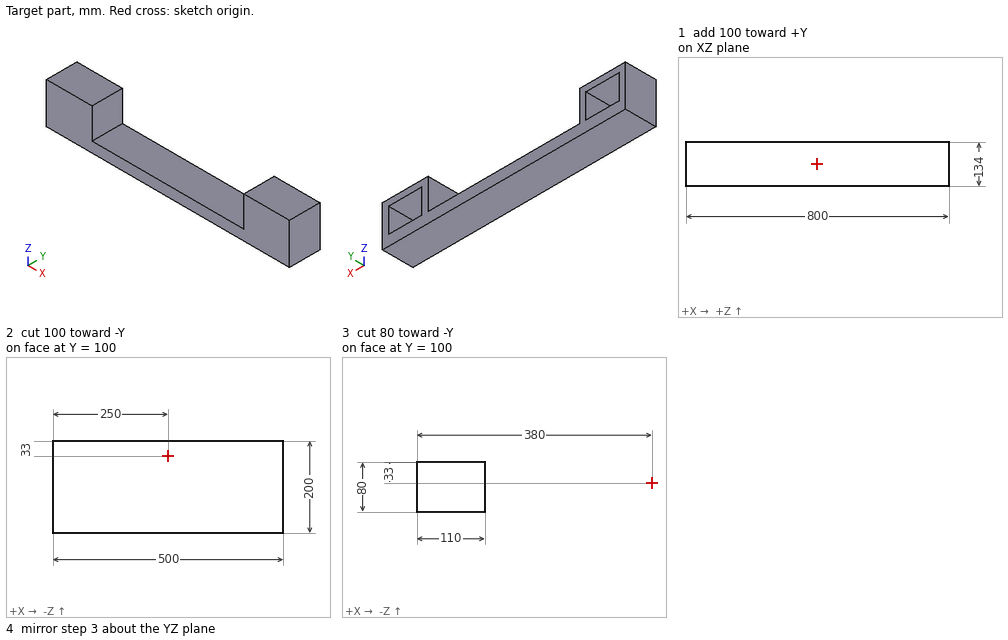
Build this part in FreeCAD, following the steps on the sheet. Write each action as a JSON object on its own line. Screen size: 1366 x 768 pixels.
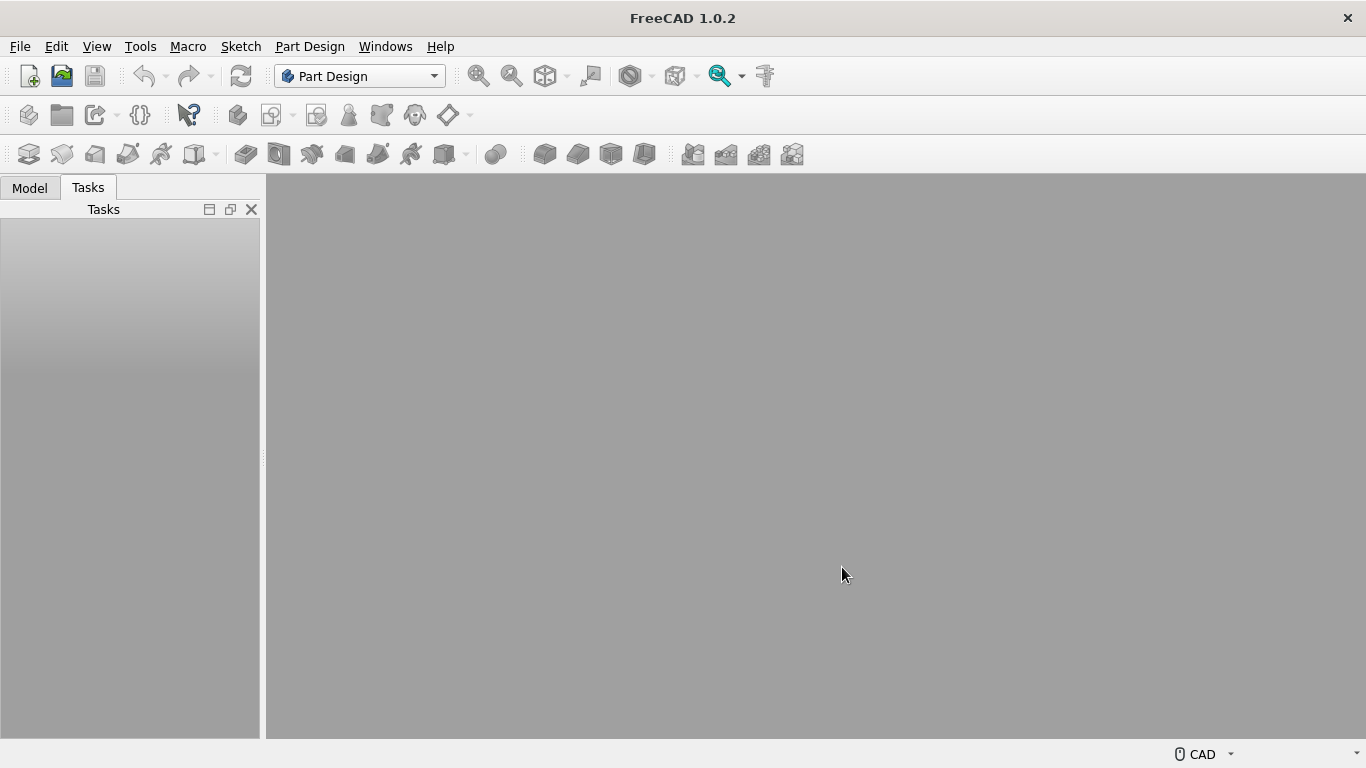
{"action": "key", "text": "ctrl+n"}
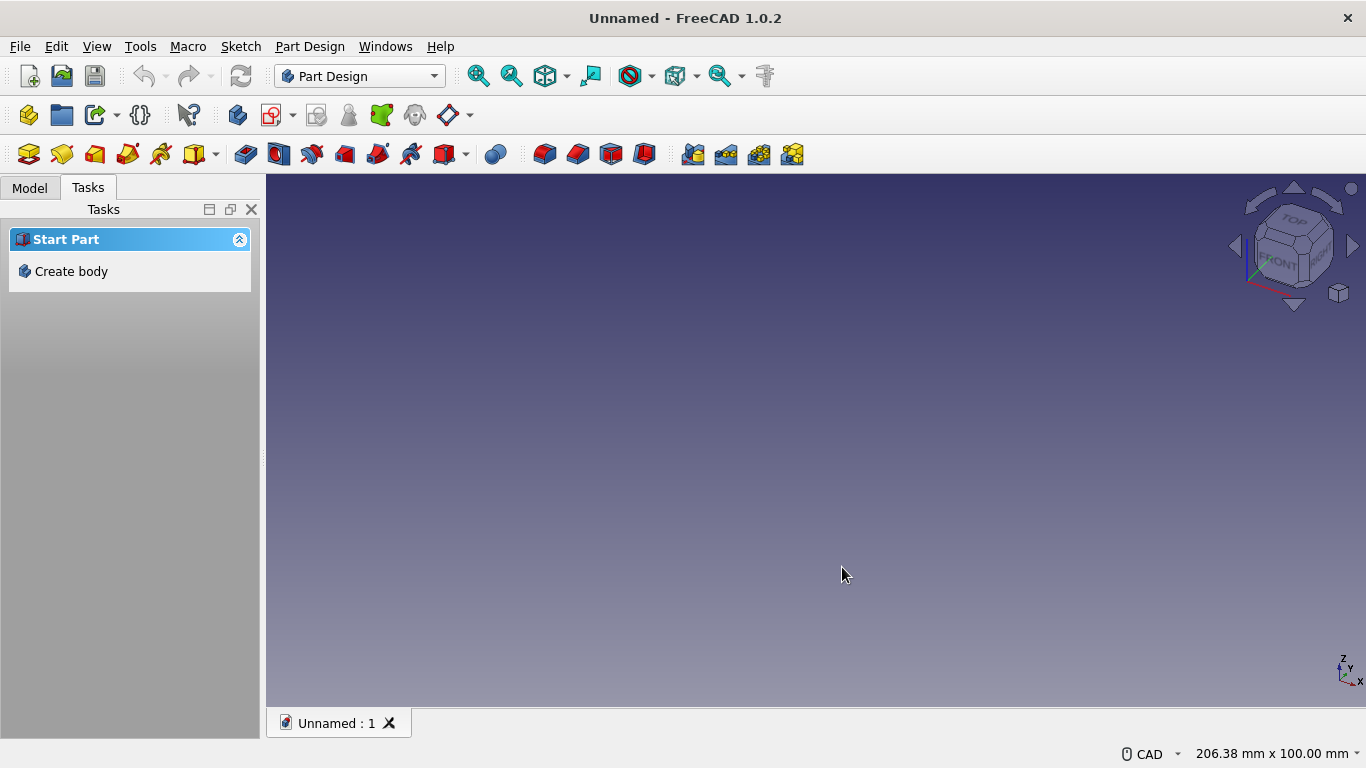
{"action": "left_click", "coordinate": [270, 116]}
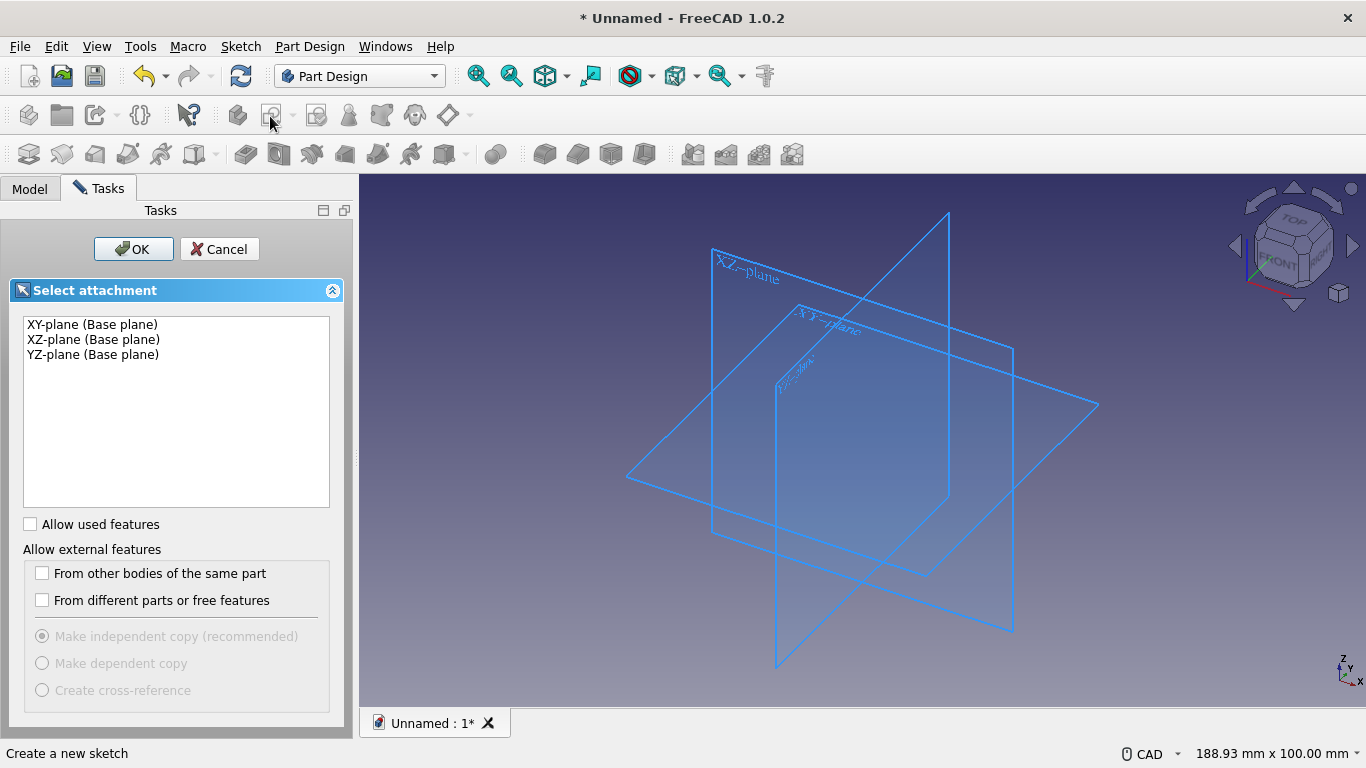
{"action": "left_click", "coordinate": [84, 340]}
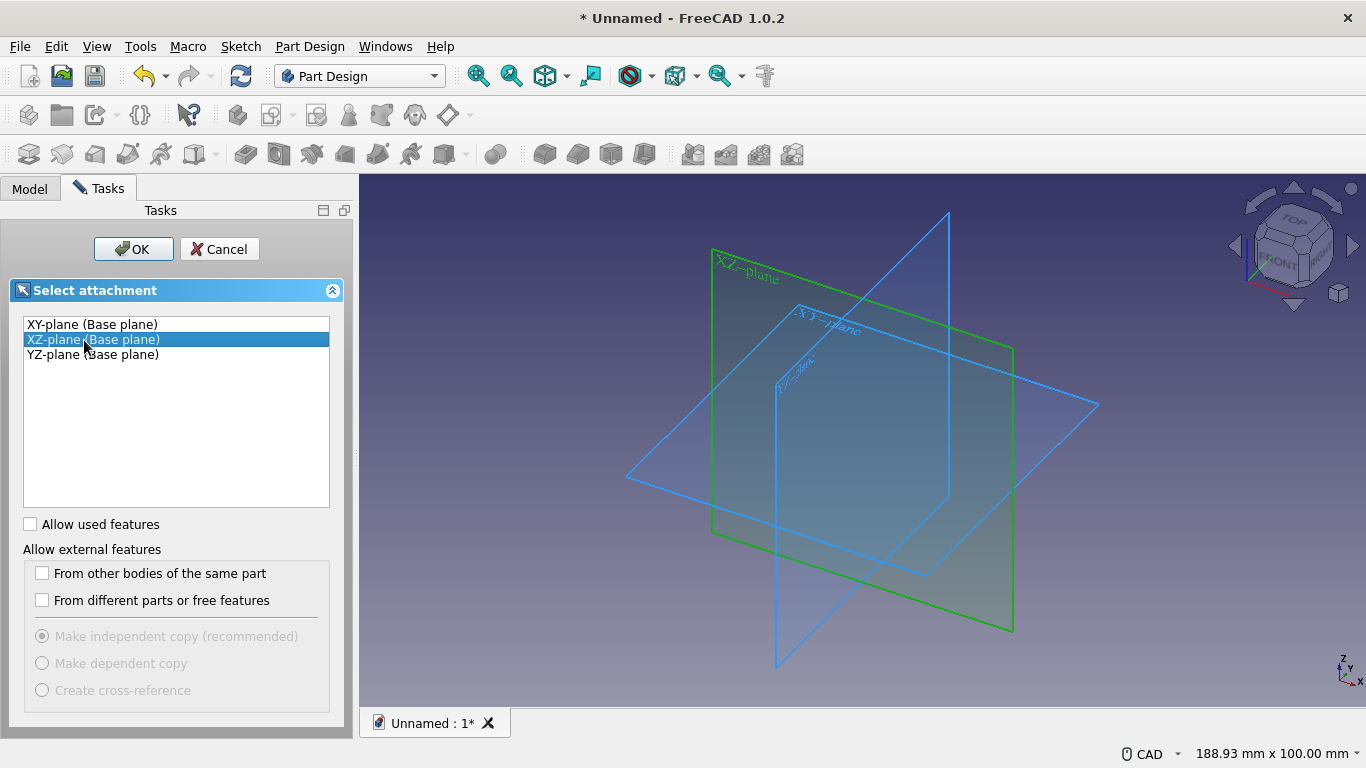
{"action": "left_click", "coordinate": [134, 249]}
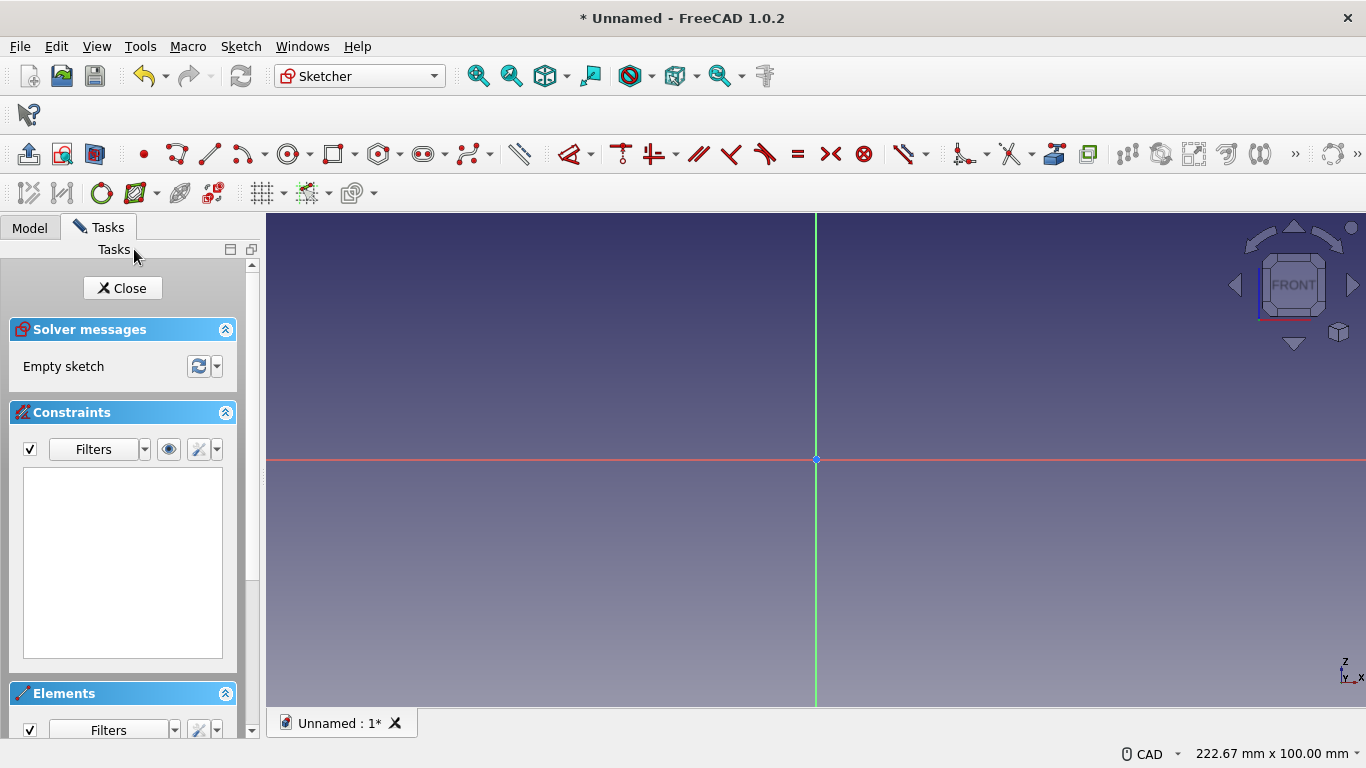
{"action": "scroll", "coordinate": [734, 460], "scroll_direction": "down", "scroll_amount": 9}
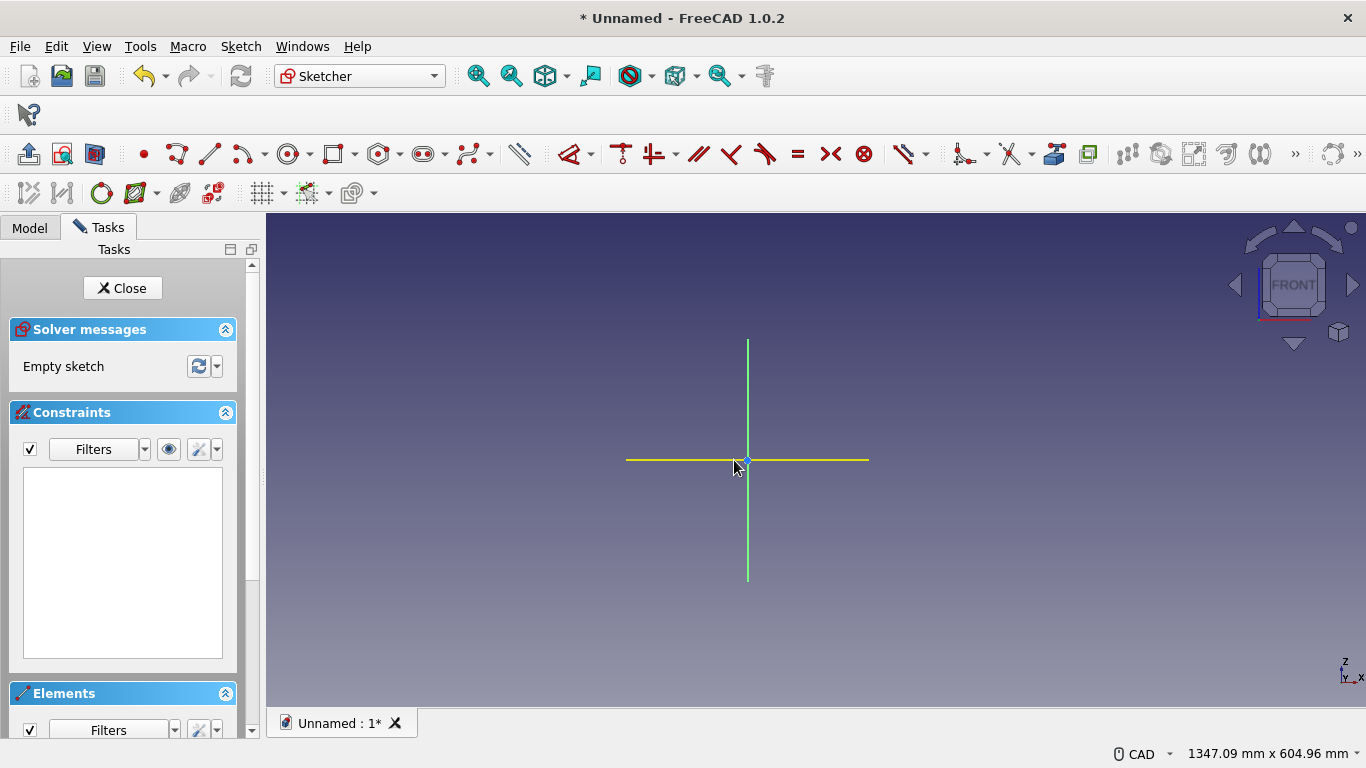
{"action": "key", "text": "g v"}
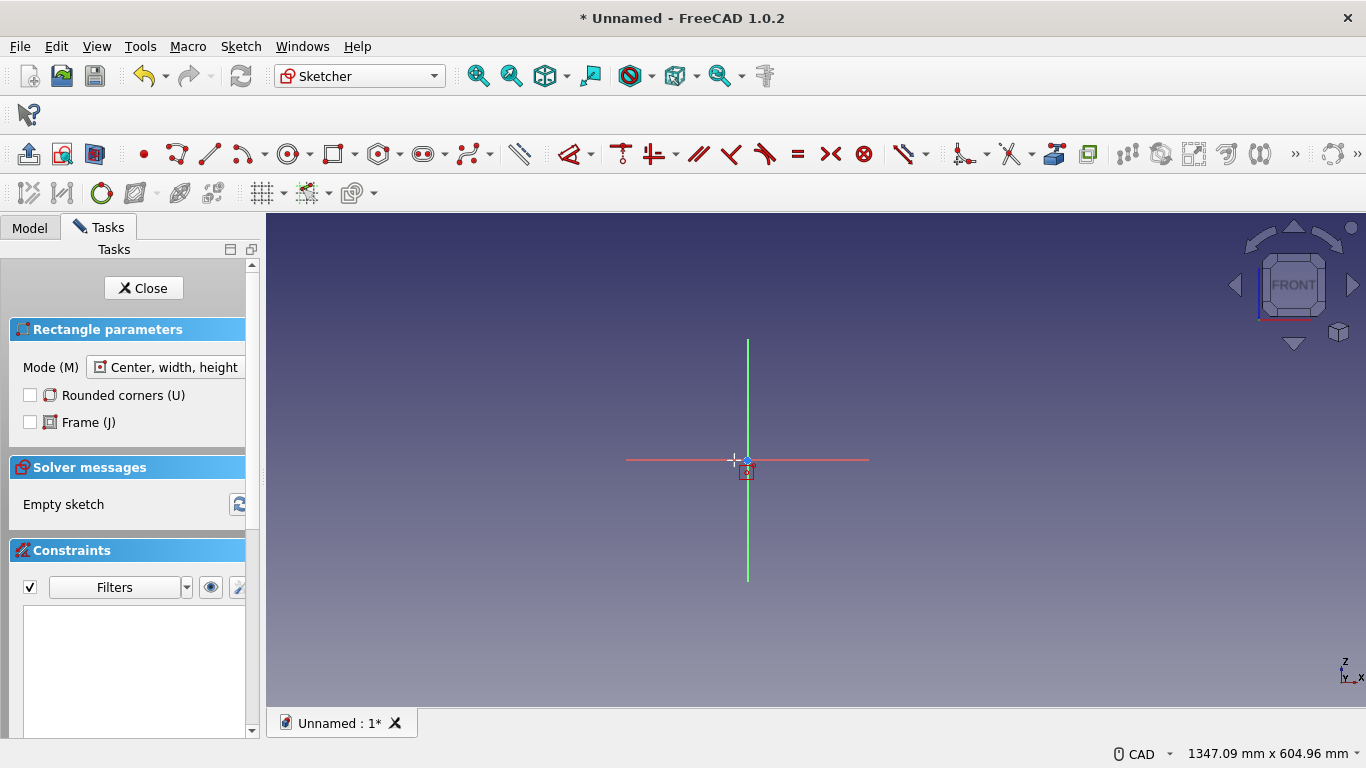
{"action": "left_click", "coordinate": [748, 460]}
{"action": "mouse_move", "coordinate": [1075, 406]}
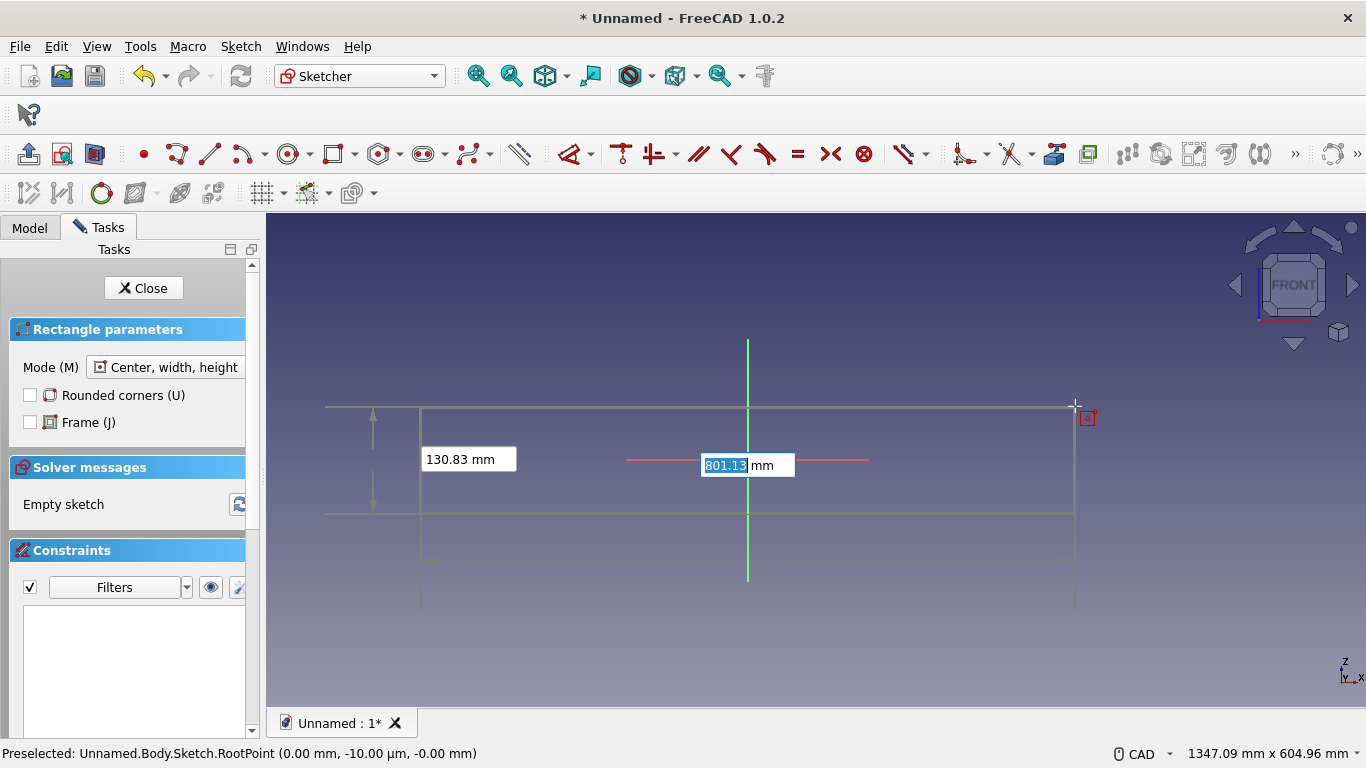
{"action": "type", "text": "800"}
{"action": "key", "text": "Tab"}
{"action": "type", "text": "134"}
{"action": "key", "text": "Return"}
{"action": "key", "text": "Escape"}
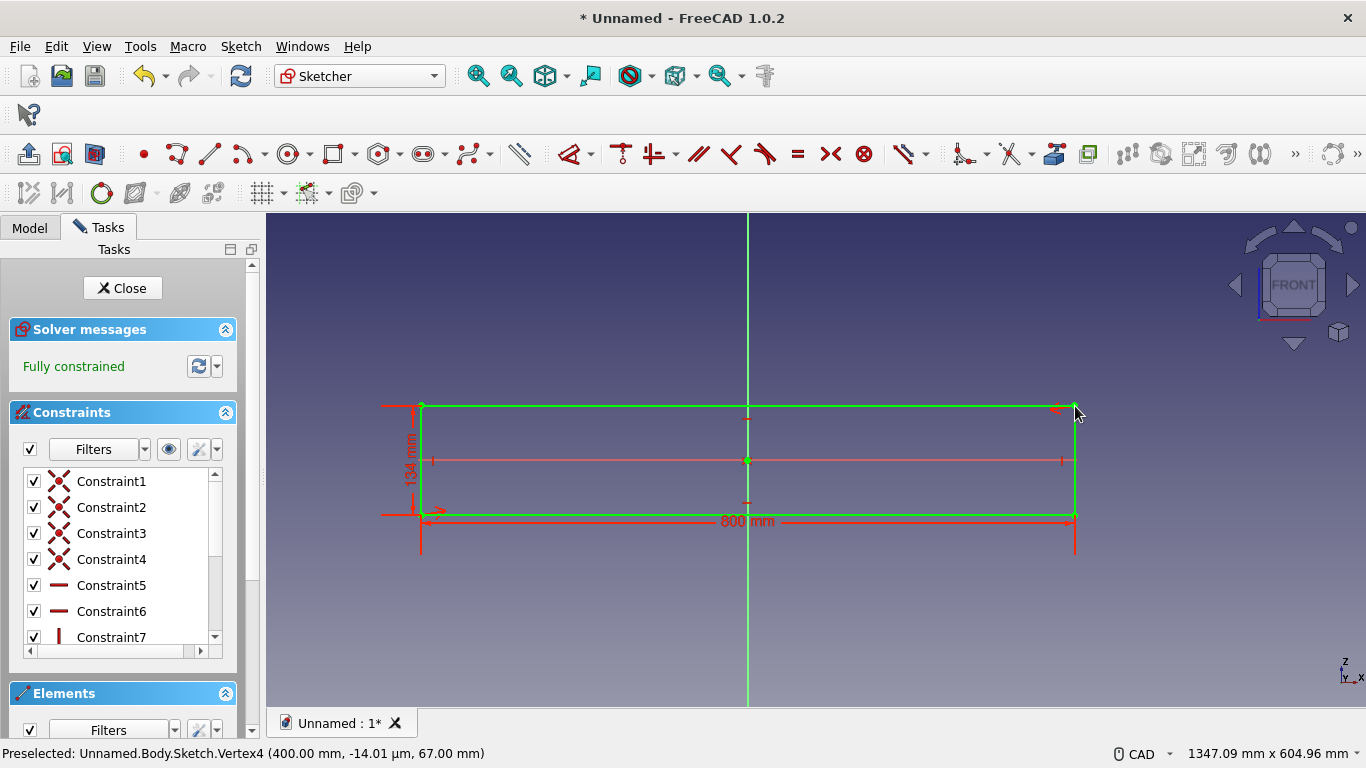
{"action": "left_click", "coordinate": [123, 288]}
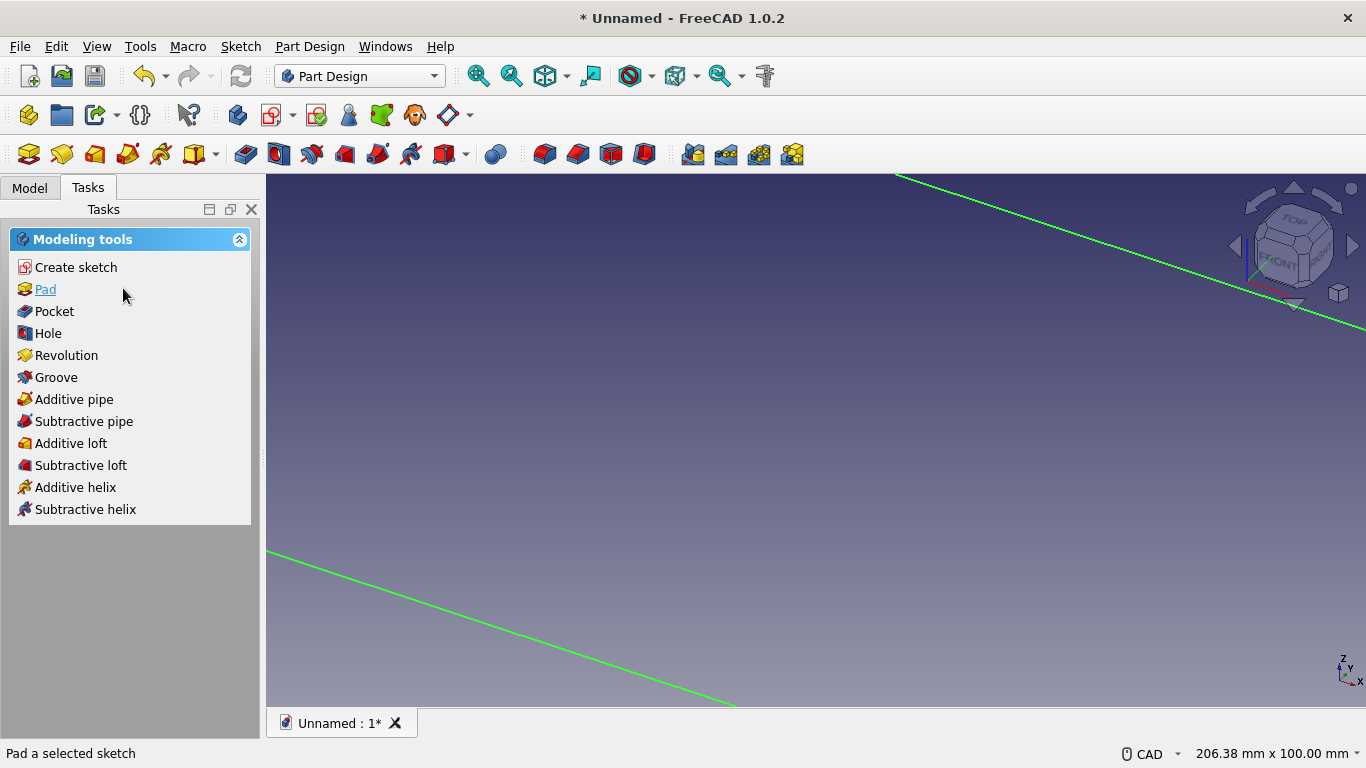
{"action": "left_click", "coordinate": [29, 154]}